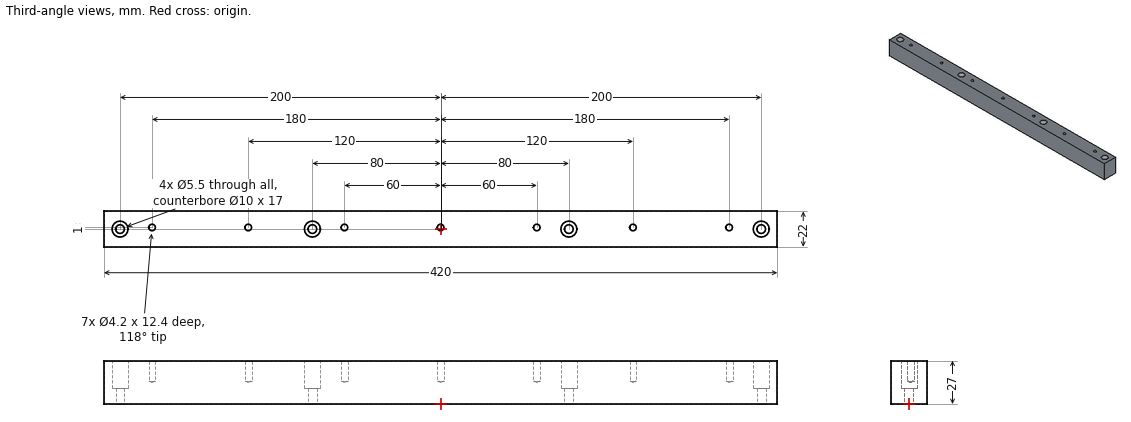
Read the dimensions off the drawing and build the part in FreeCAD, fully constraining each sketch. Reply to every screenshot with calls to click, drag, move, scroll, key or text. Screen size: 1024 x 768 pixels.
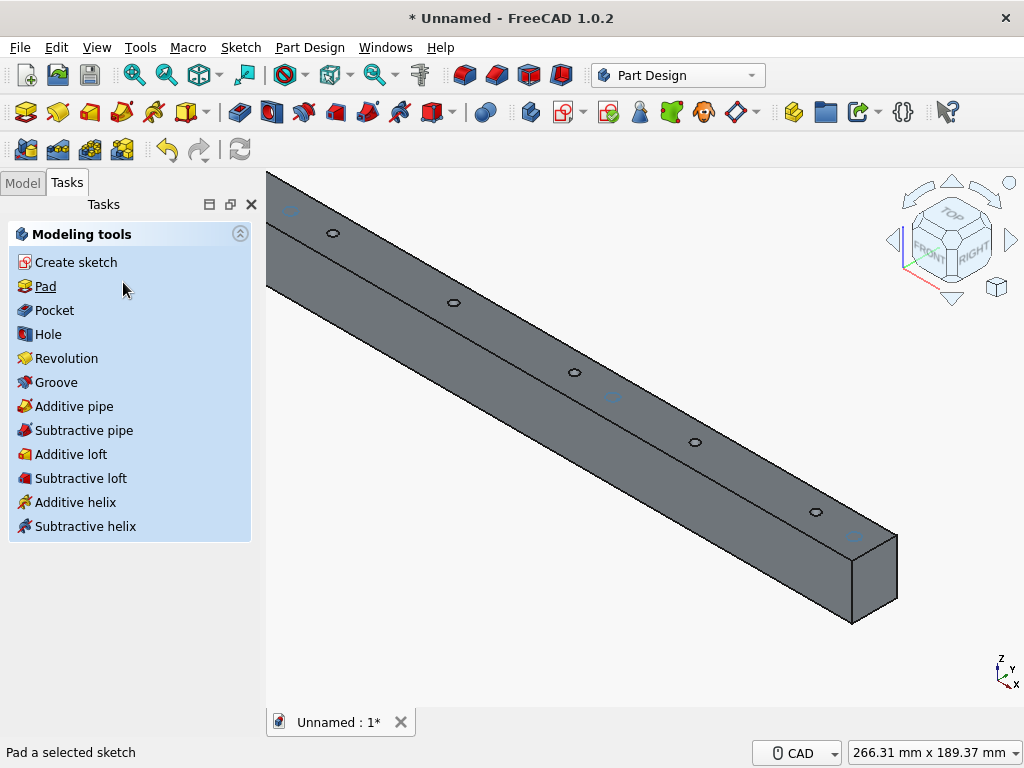
click(272, 112)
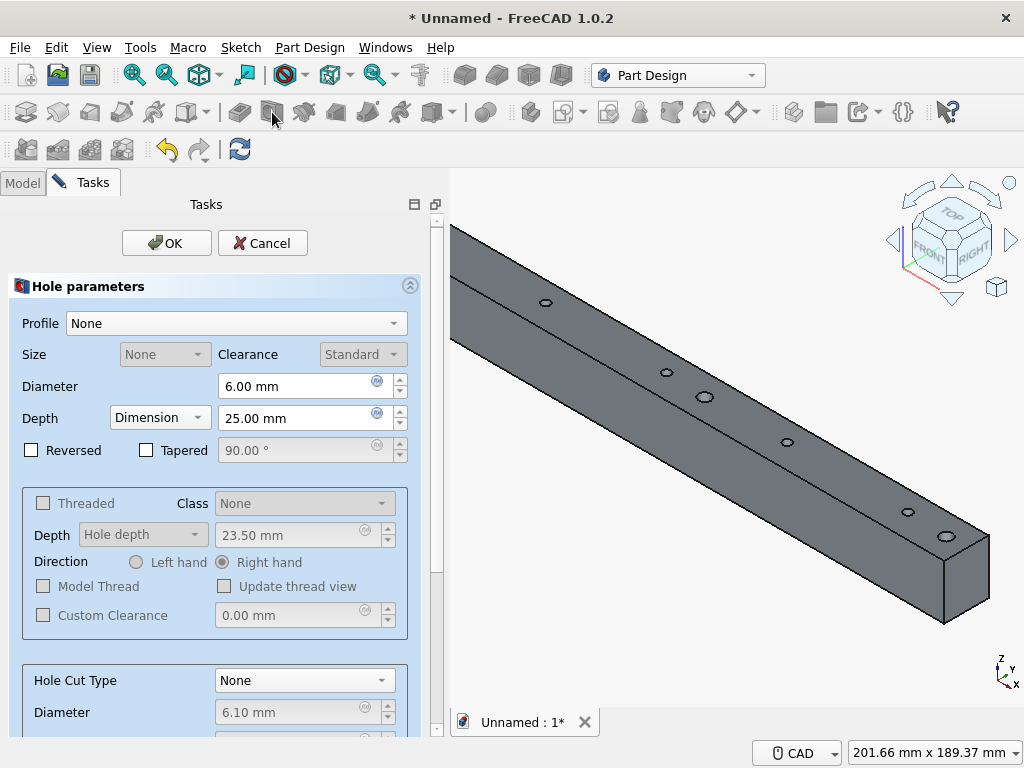
triple_click(305, 386)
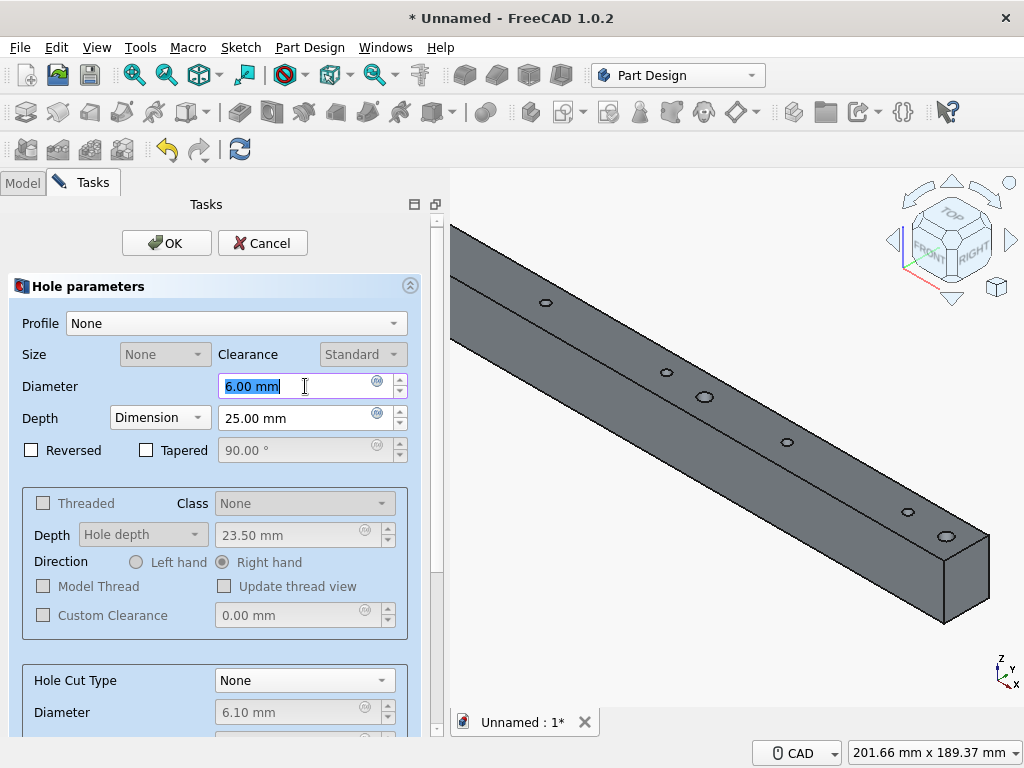
text(5.5)
key(Tab)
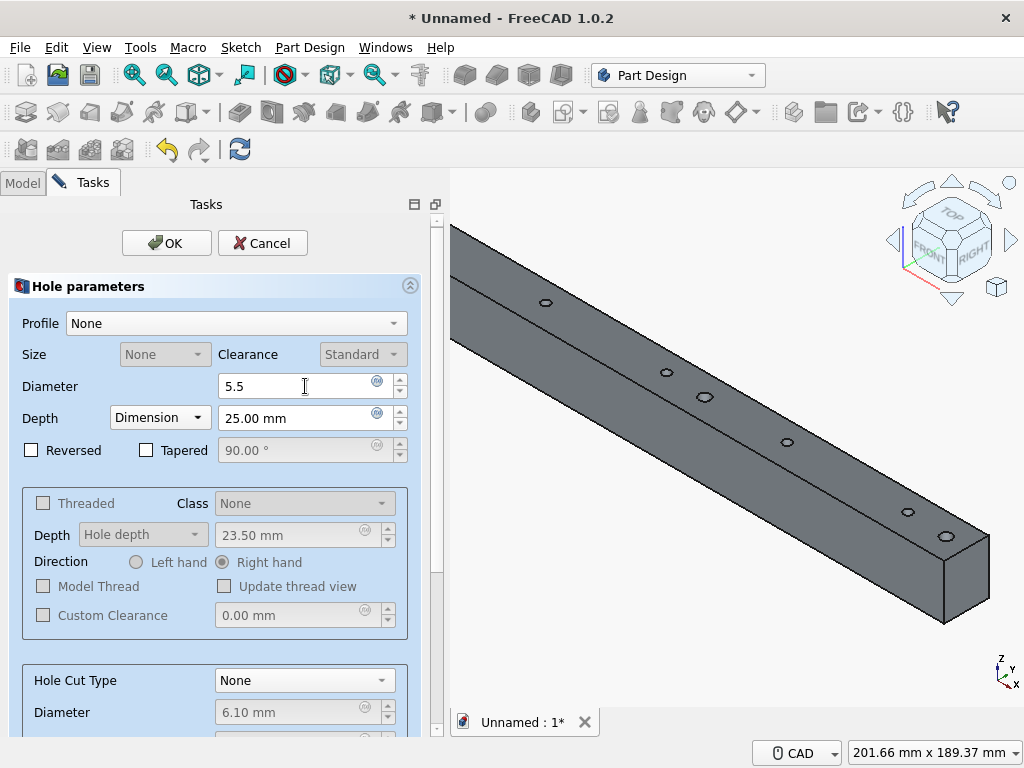
click(161, 418)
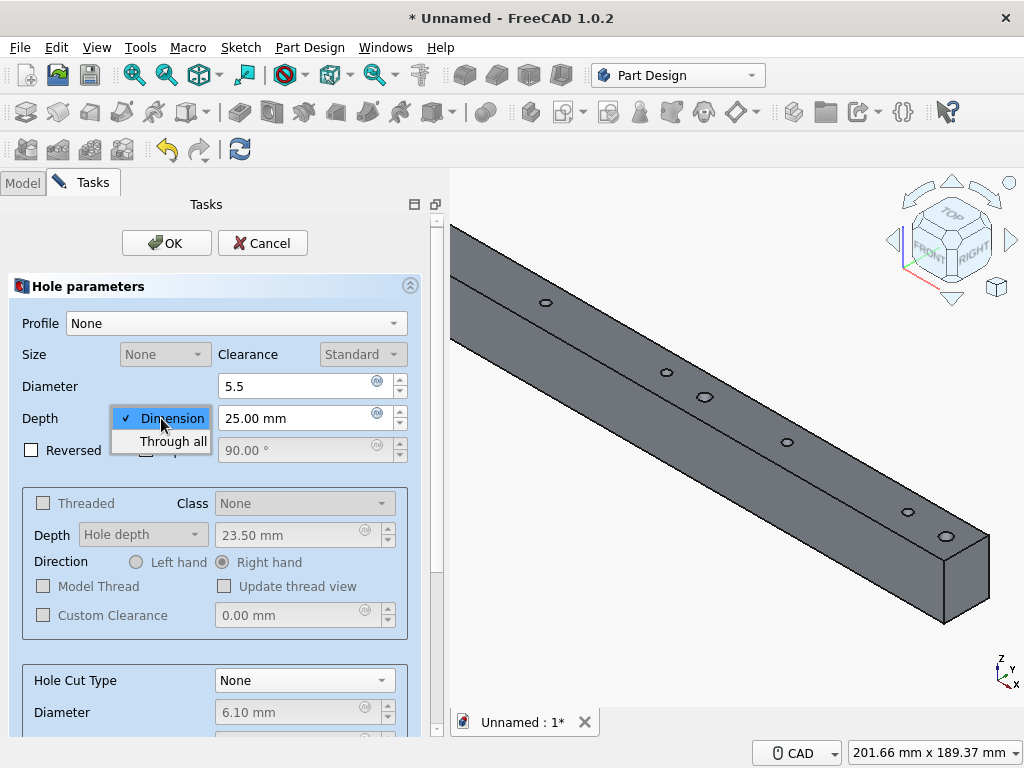
click(160, 442)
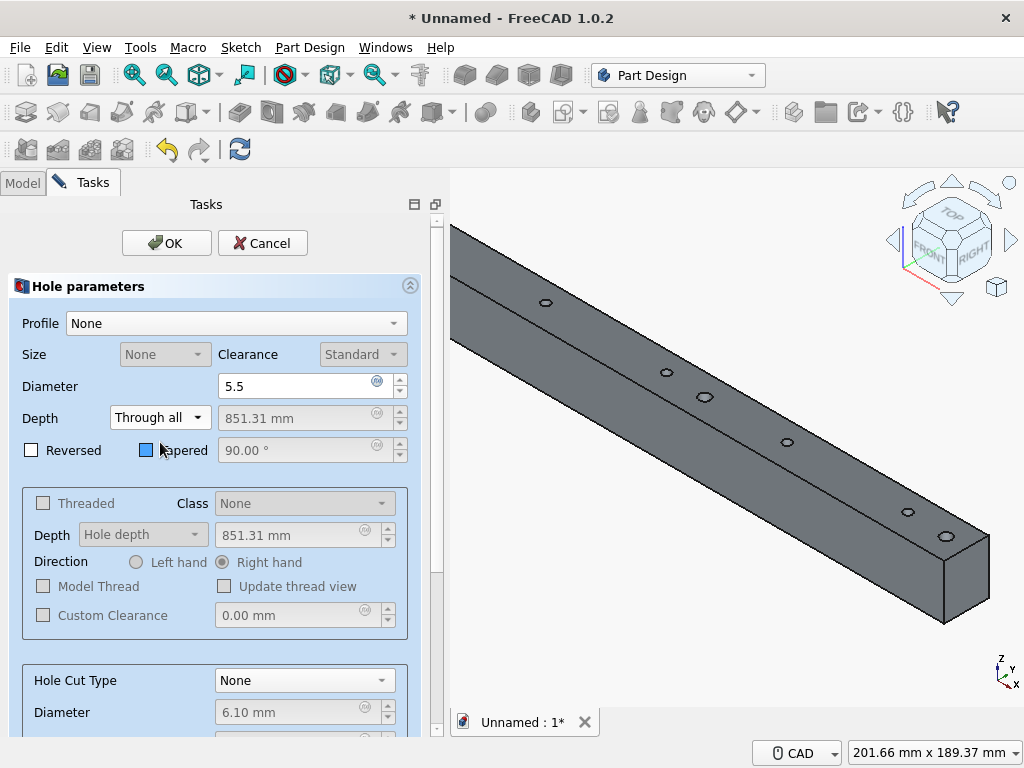
click(306, 680)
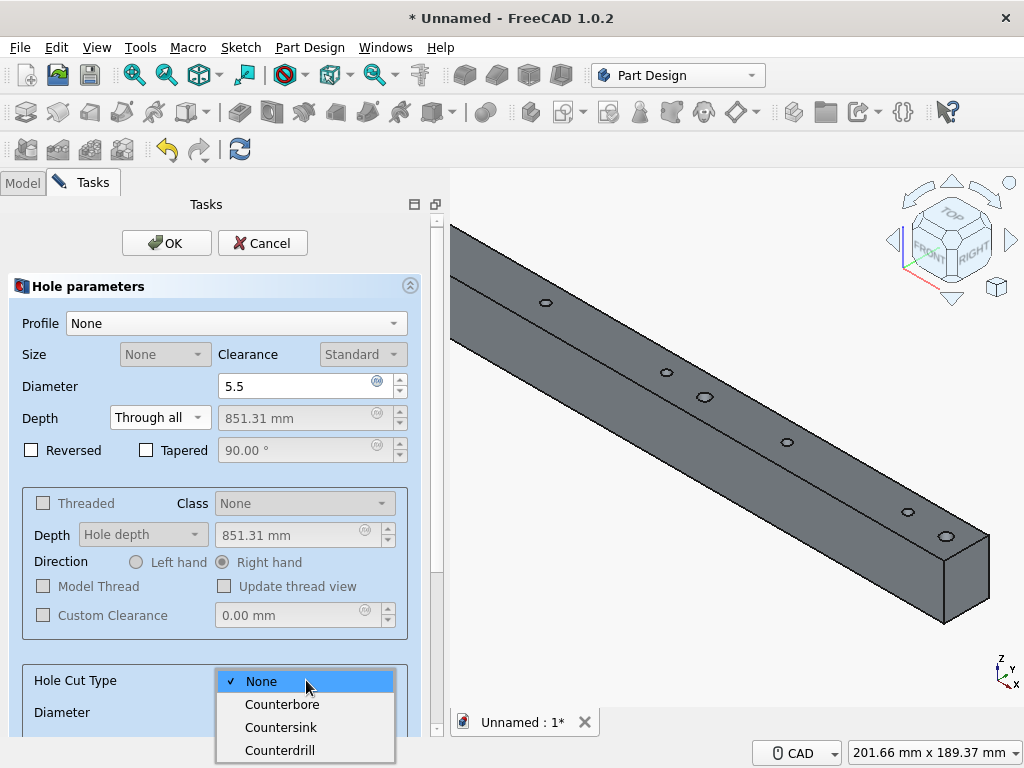
click(304, 704)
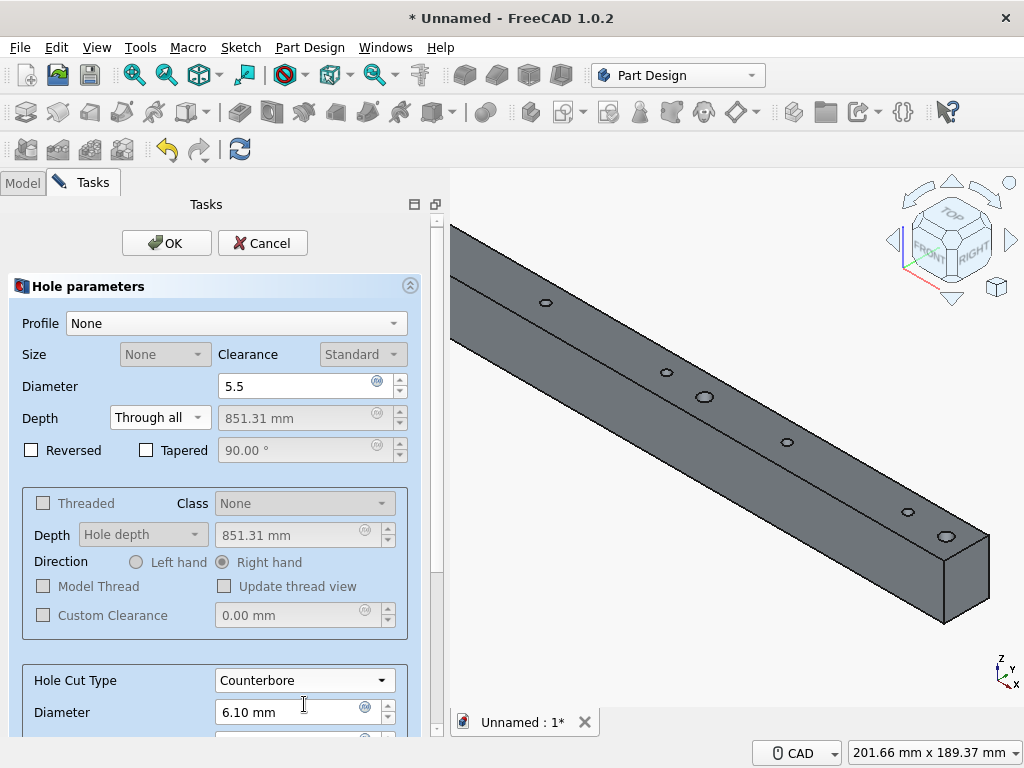
triple_click(298, 712)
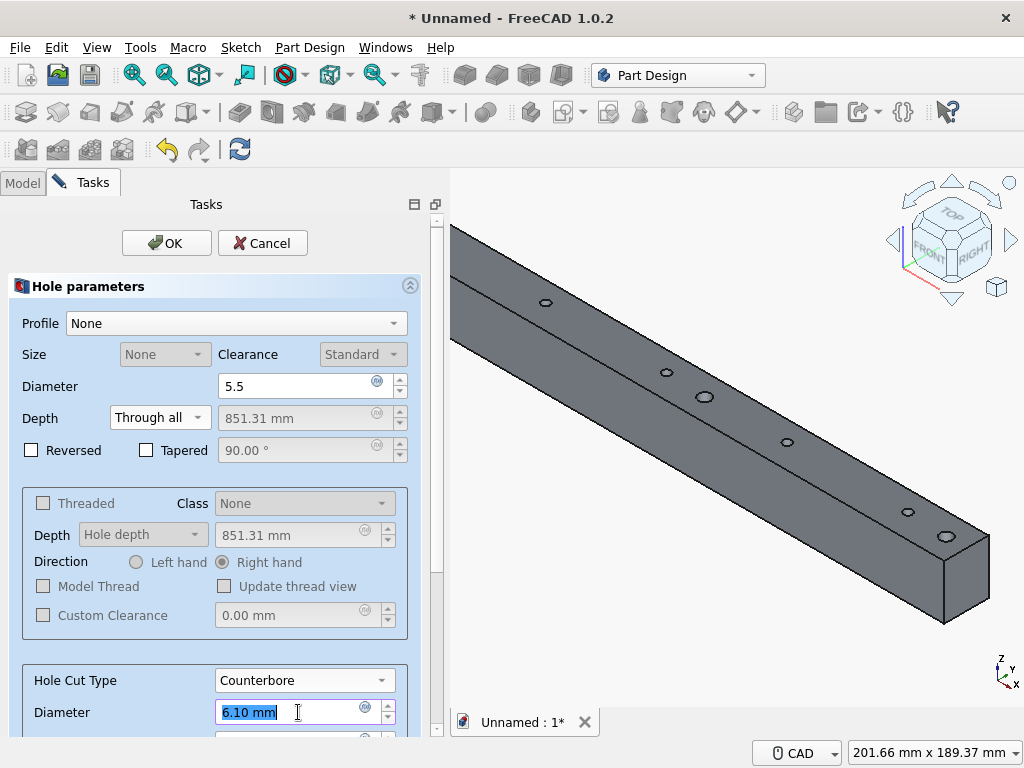
text(10)
key(Tab)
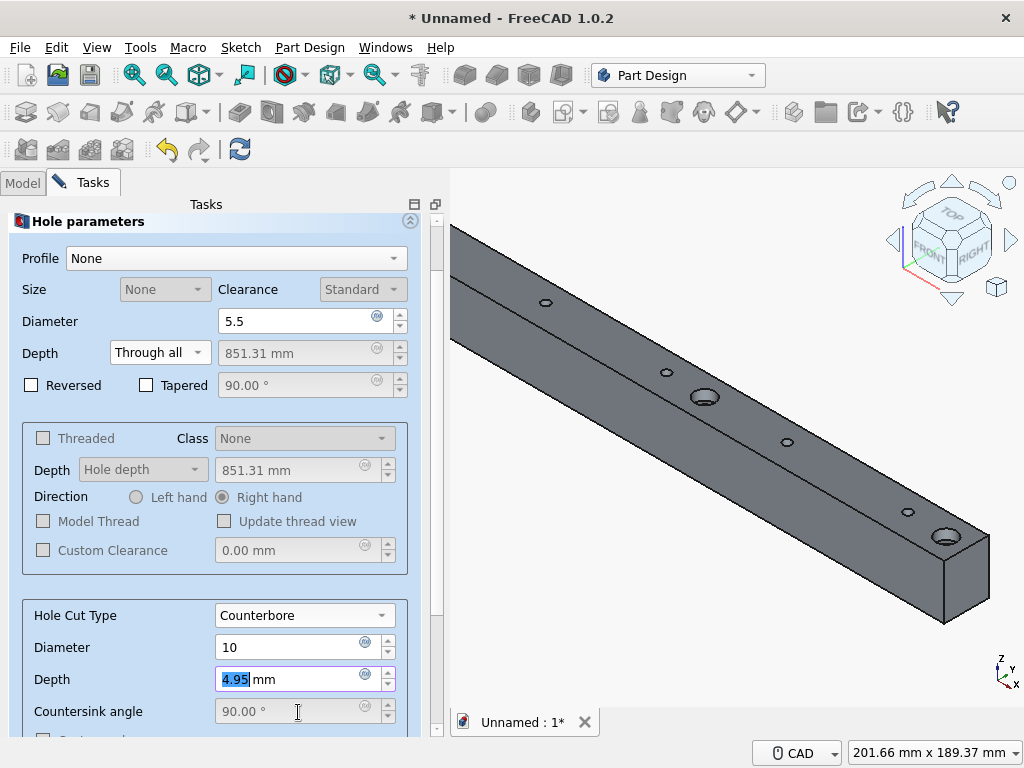
text(17)
key(Tab)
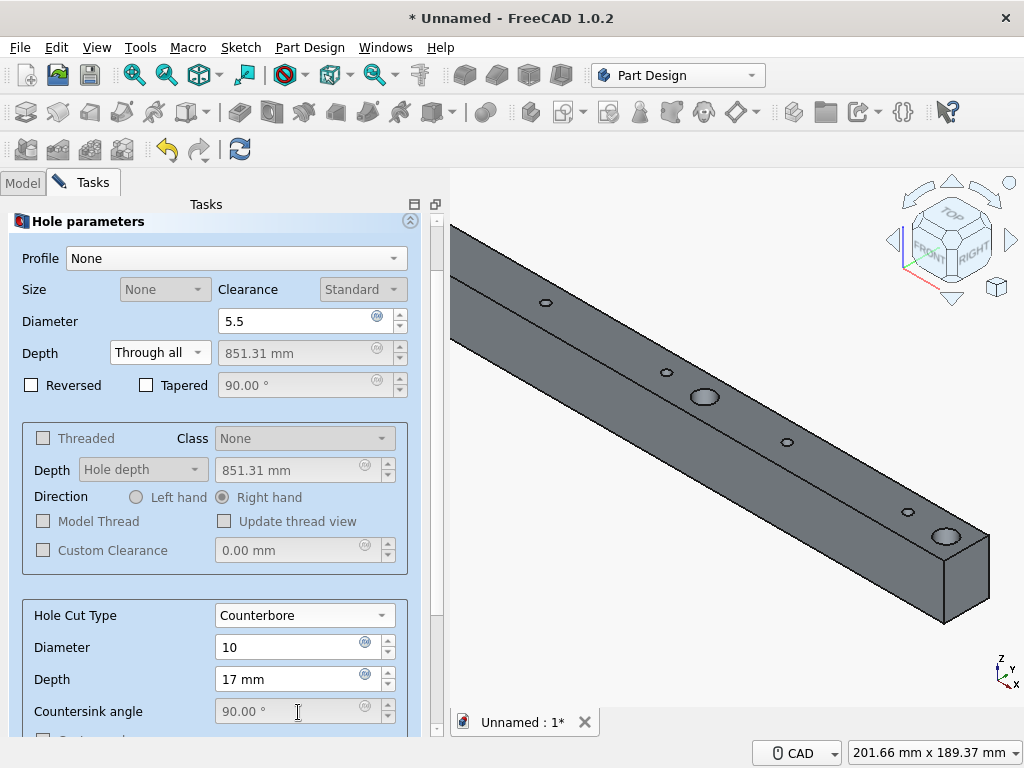
scroll(437, 475, up, 2)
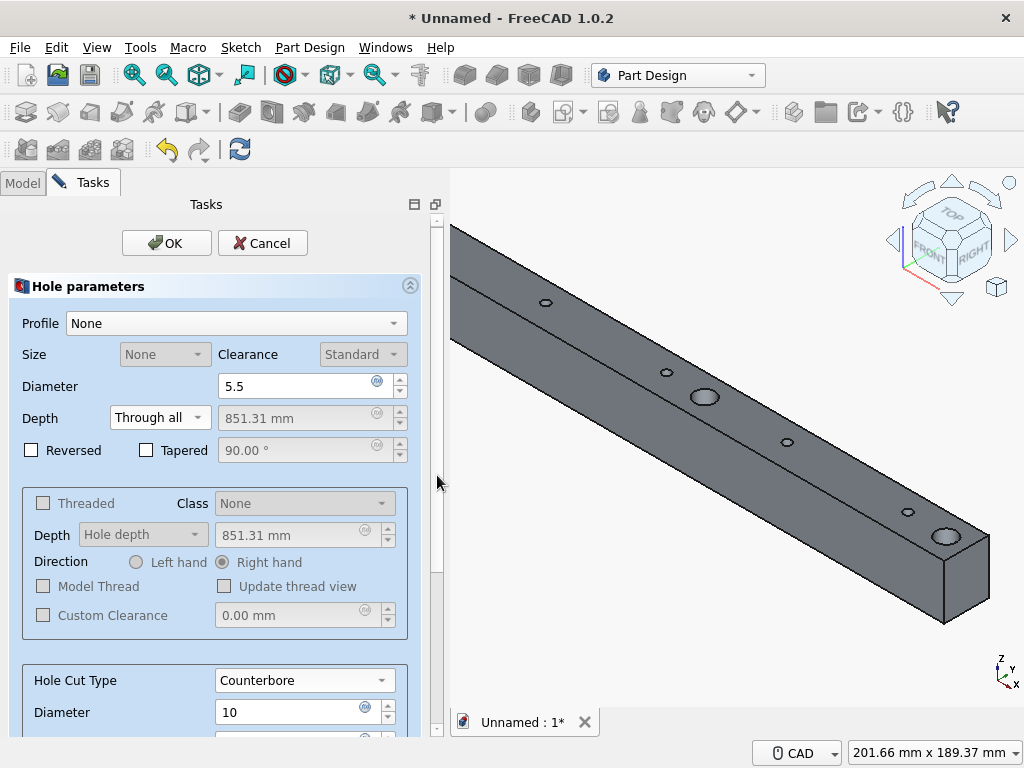
click(167, 243)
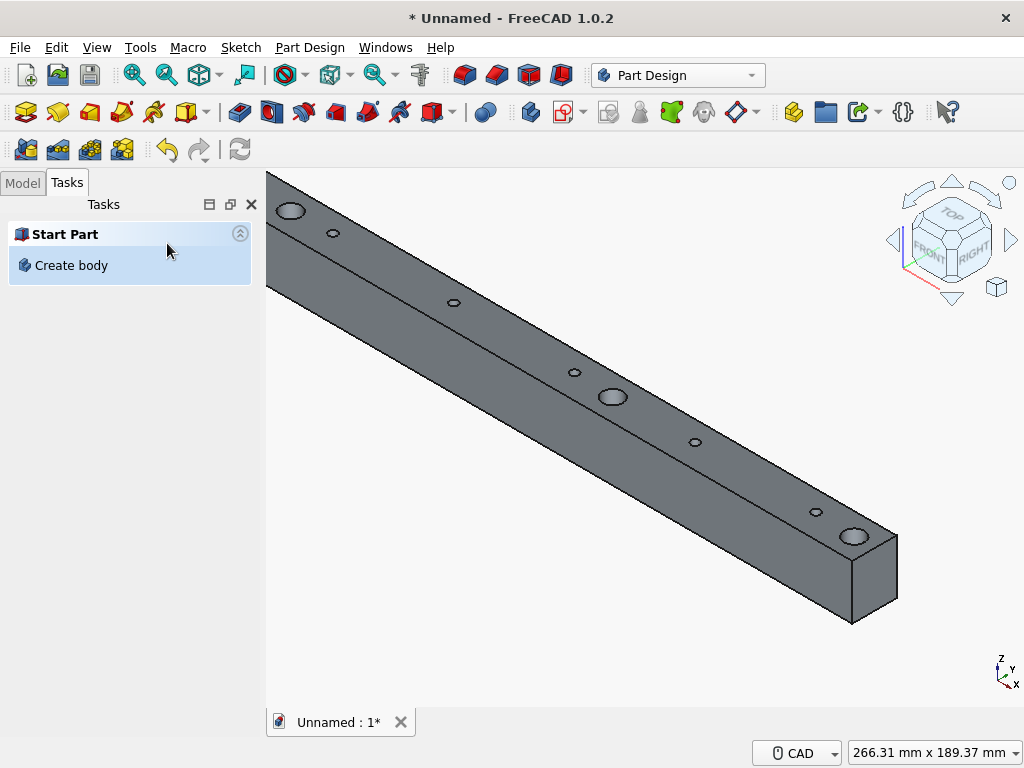
key(v)
key(f)